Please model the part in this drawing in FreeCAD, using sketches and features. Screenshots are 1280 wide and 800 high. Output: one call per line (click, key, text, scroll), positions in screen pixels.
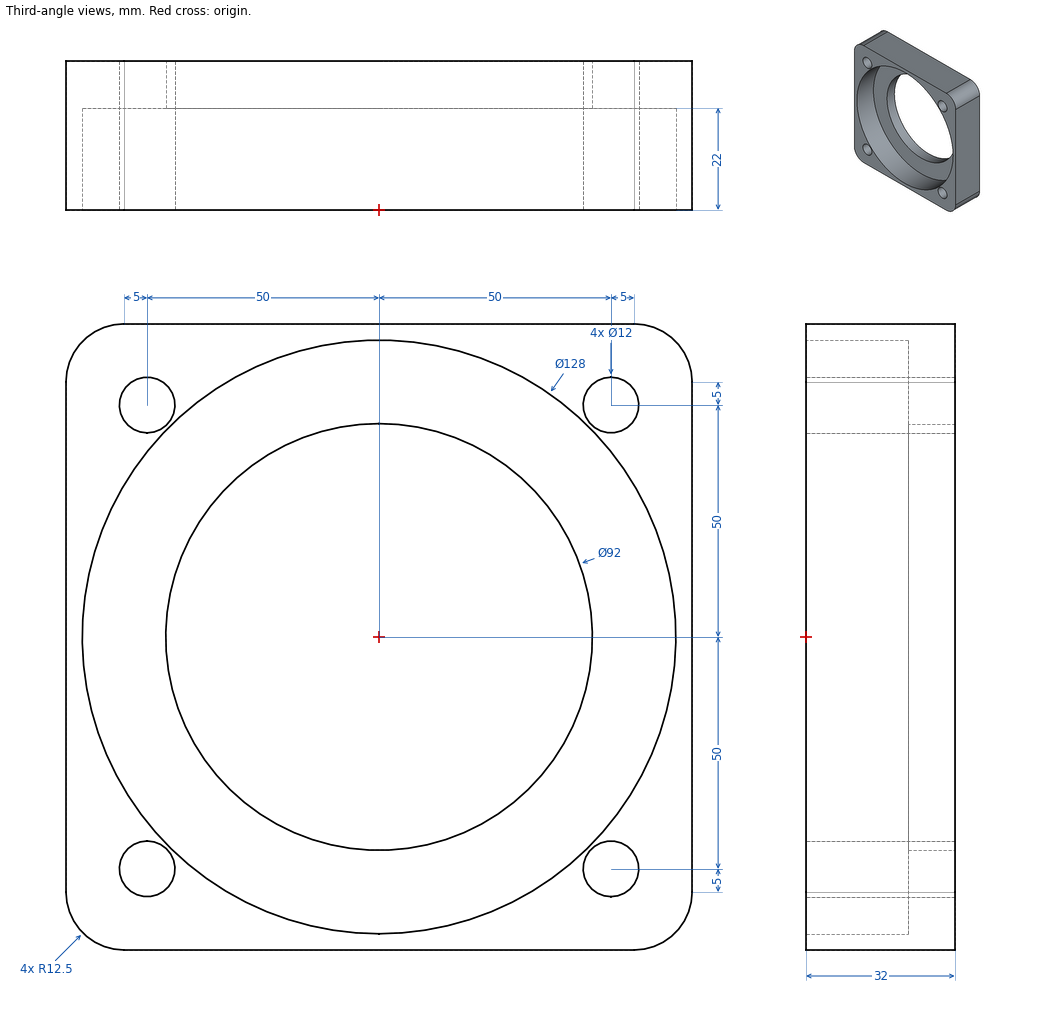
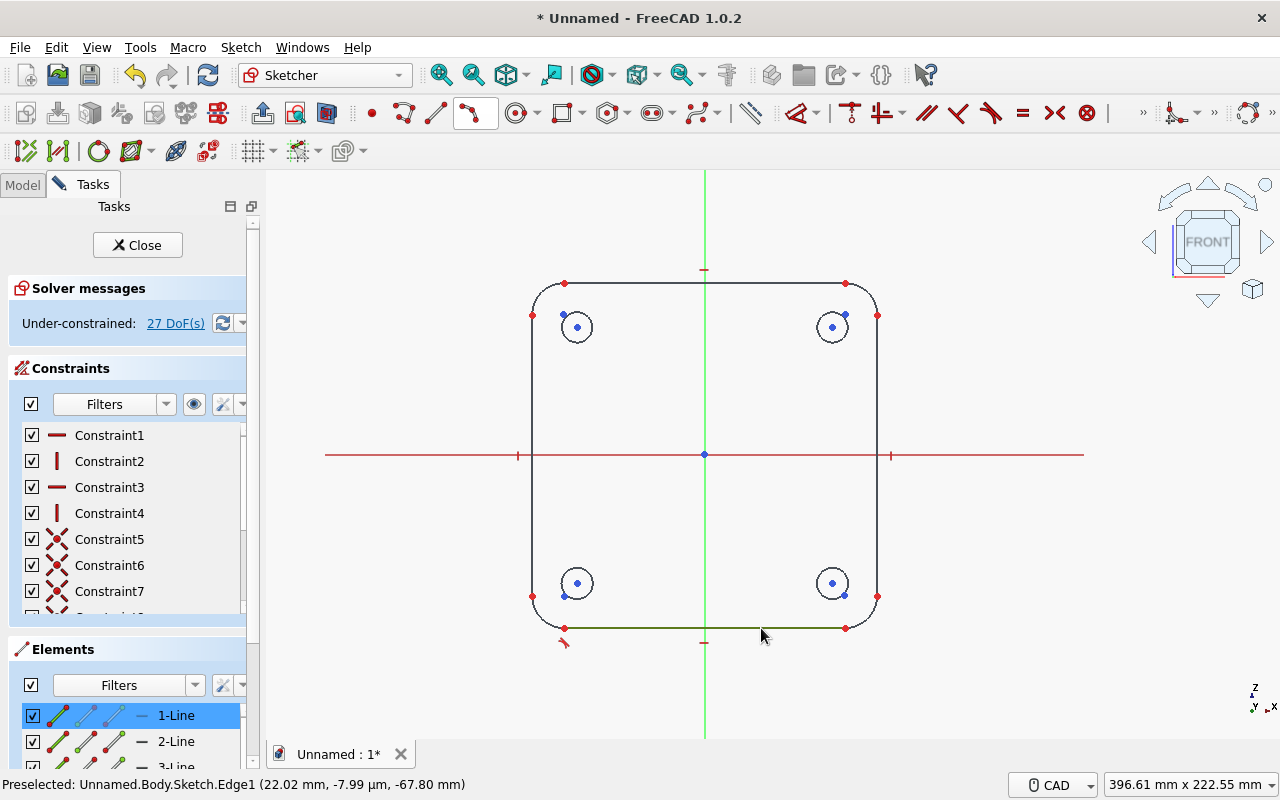
click(860, 624)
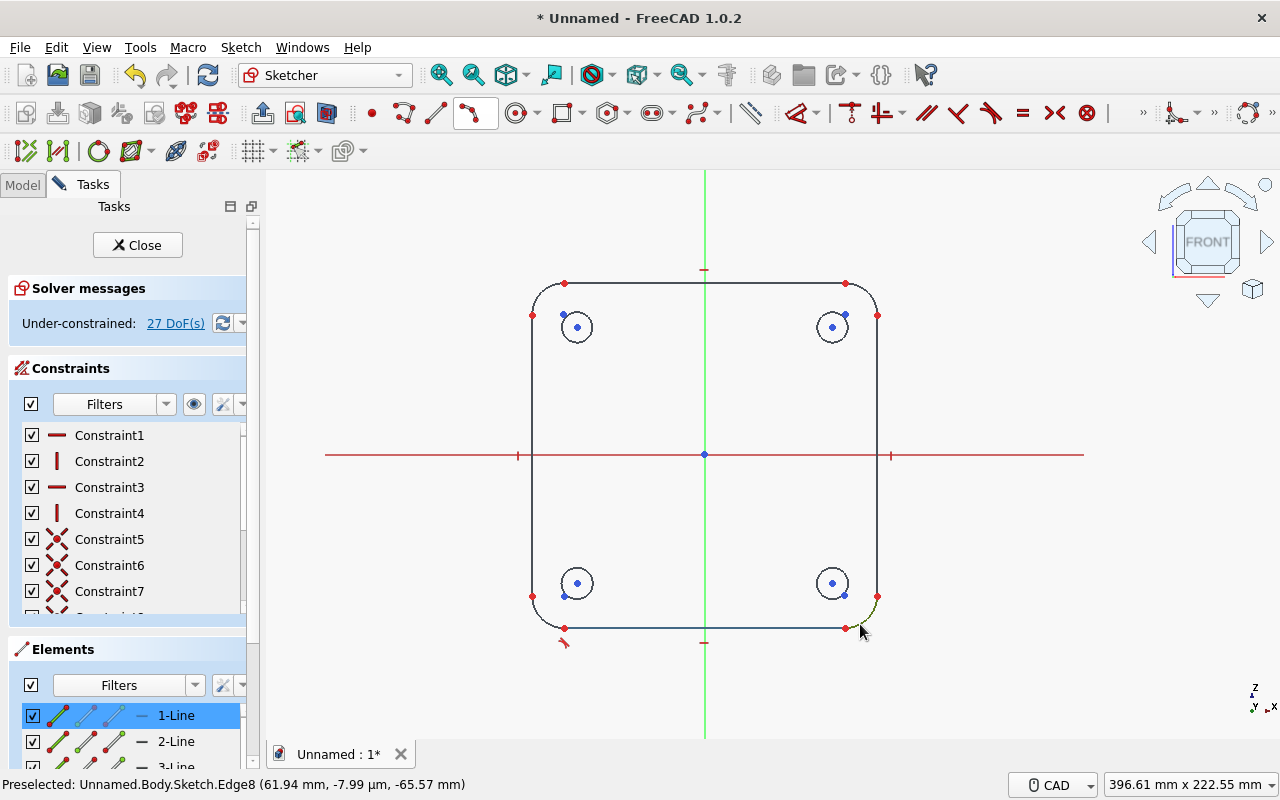
click(992, 114)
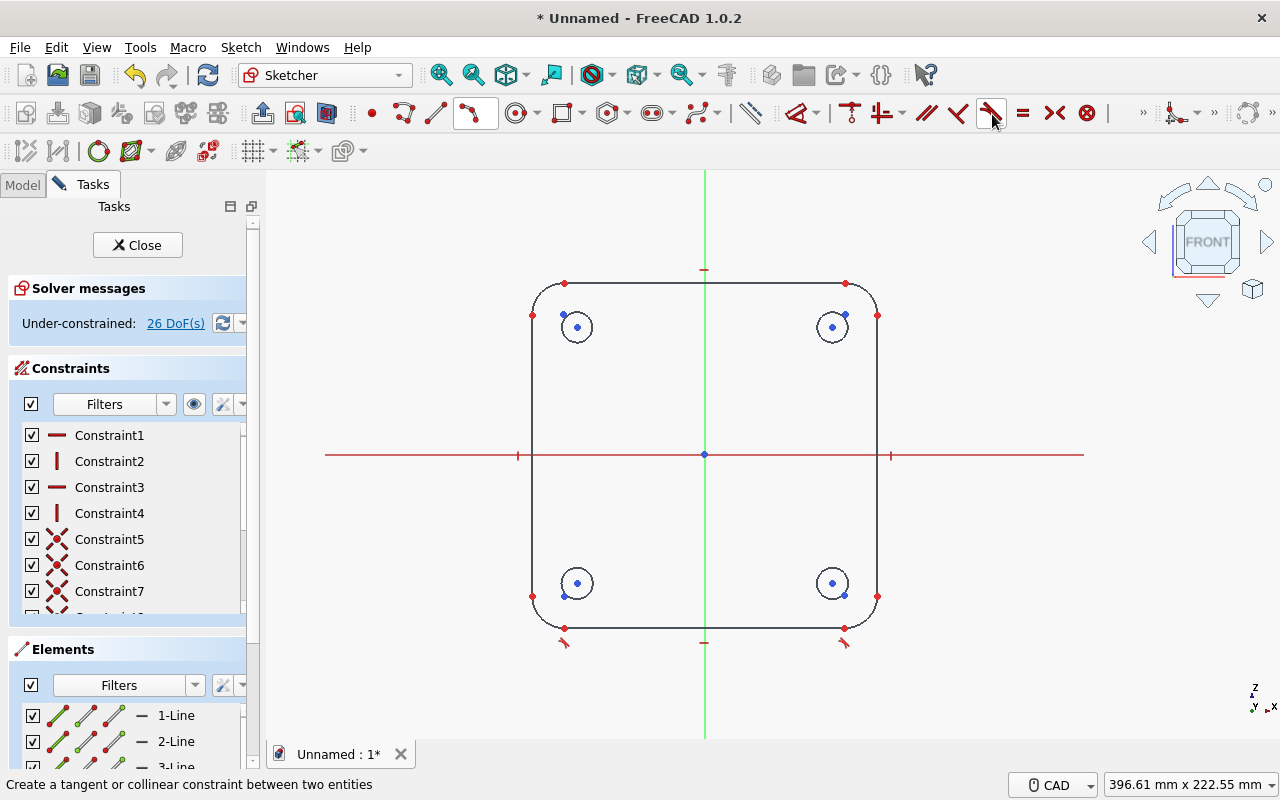
click(532, 512)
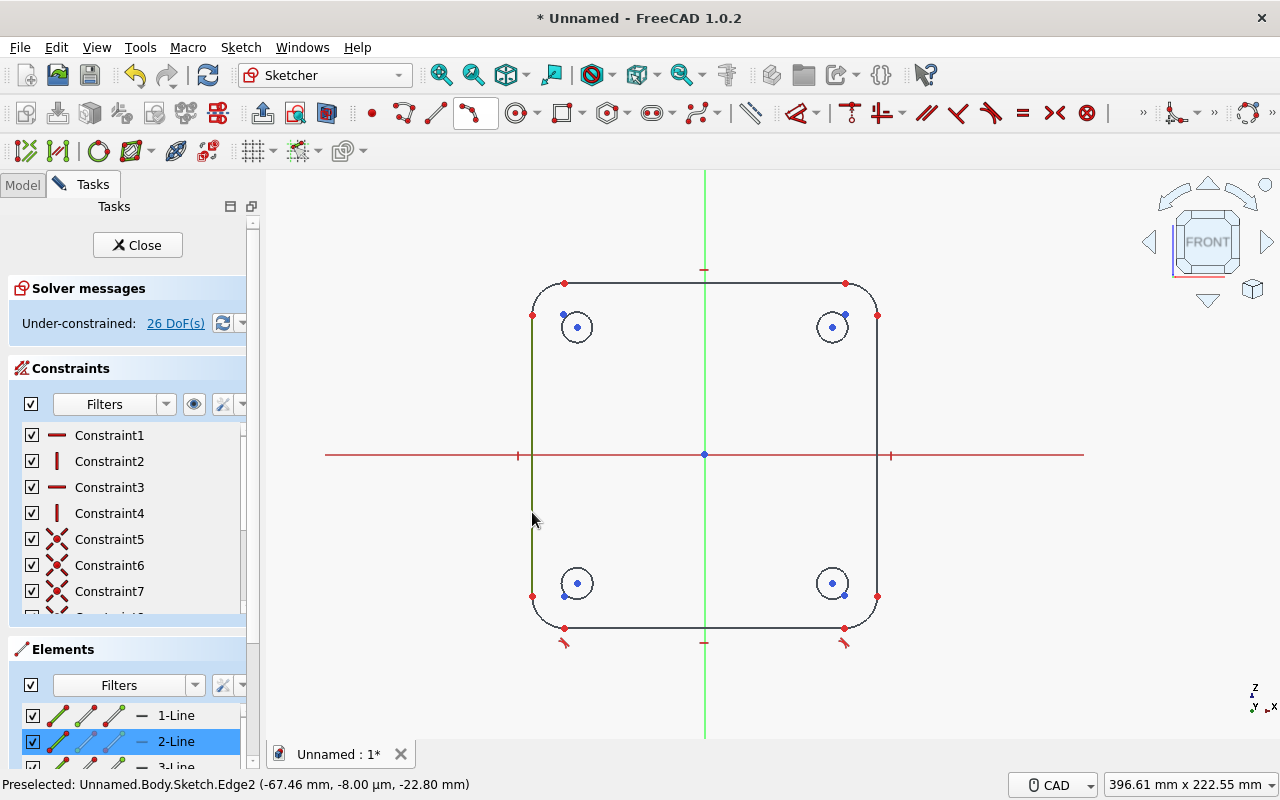
click(536, 611)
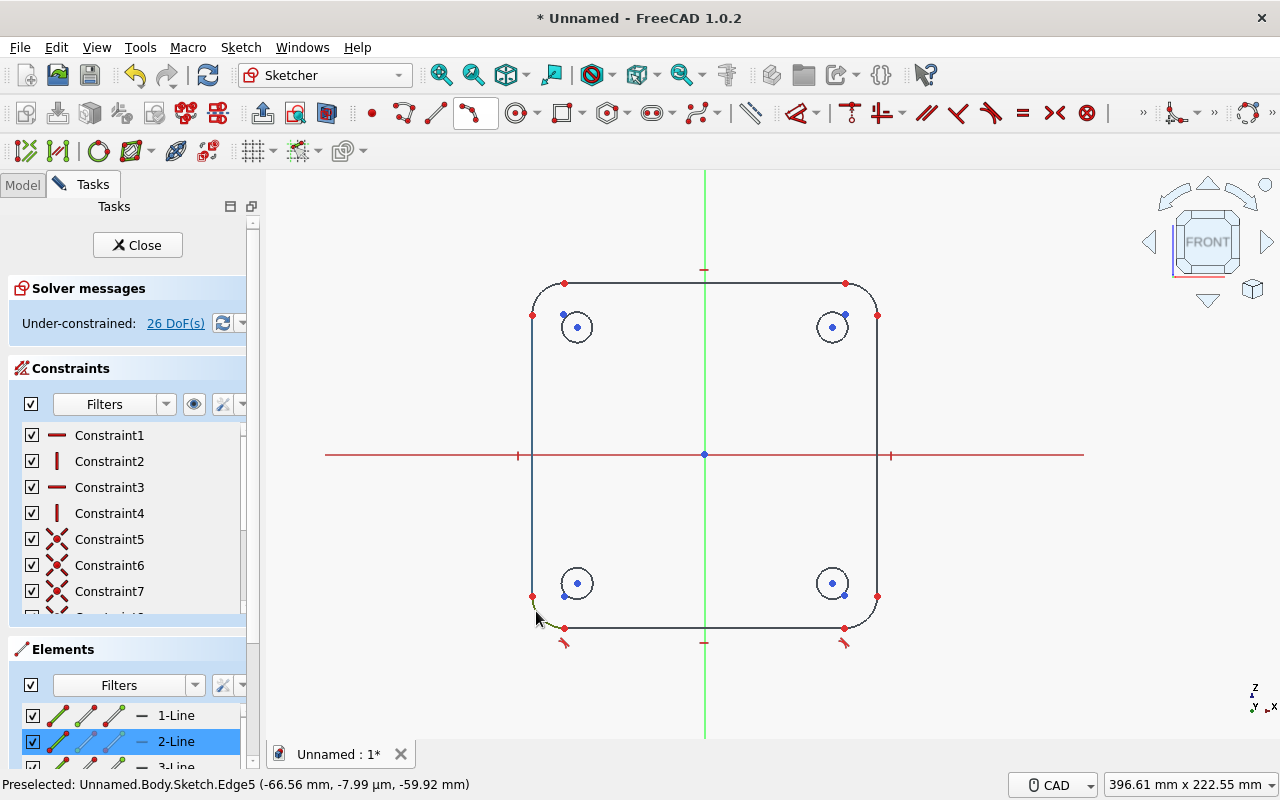
click(992, 114)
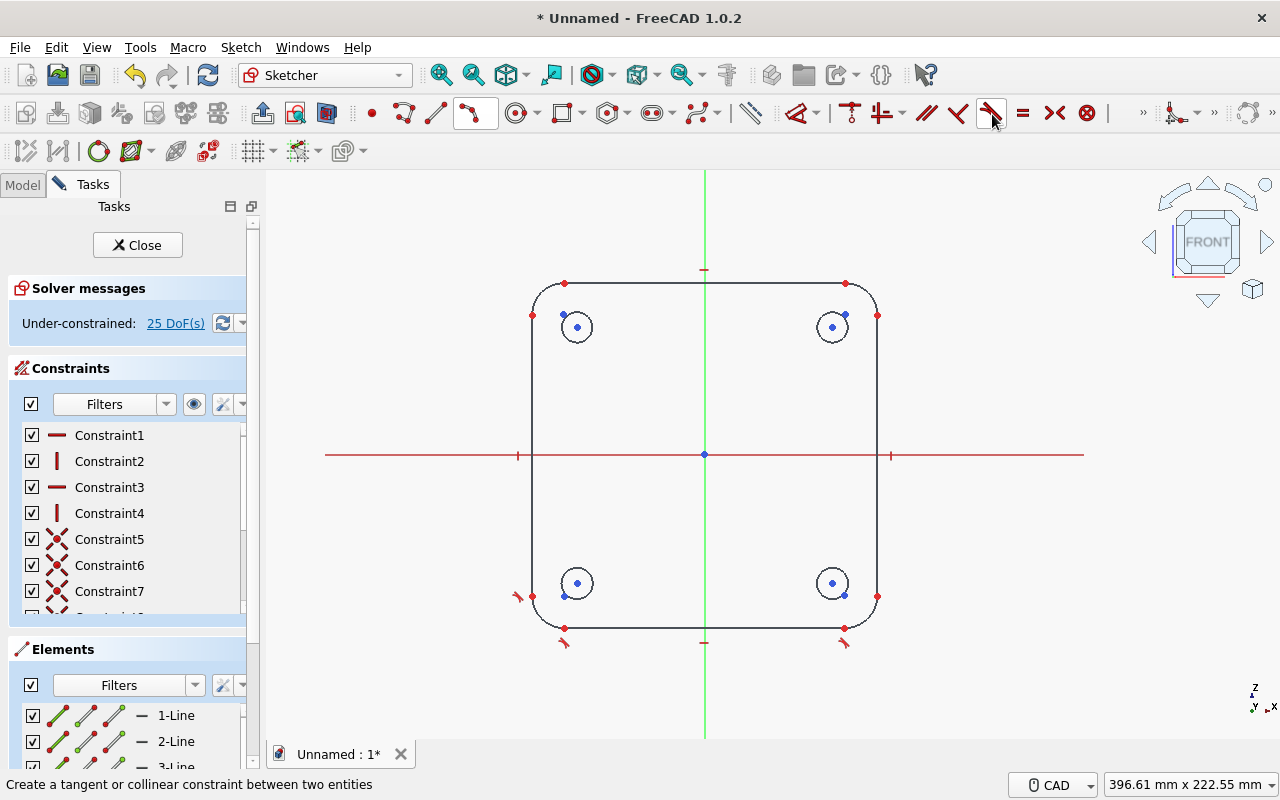
click(532, 512)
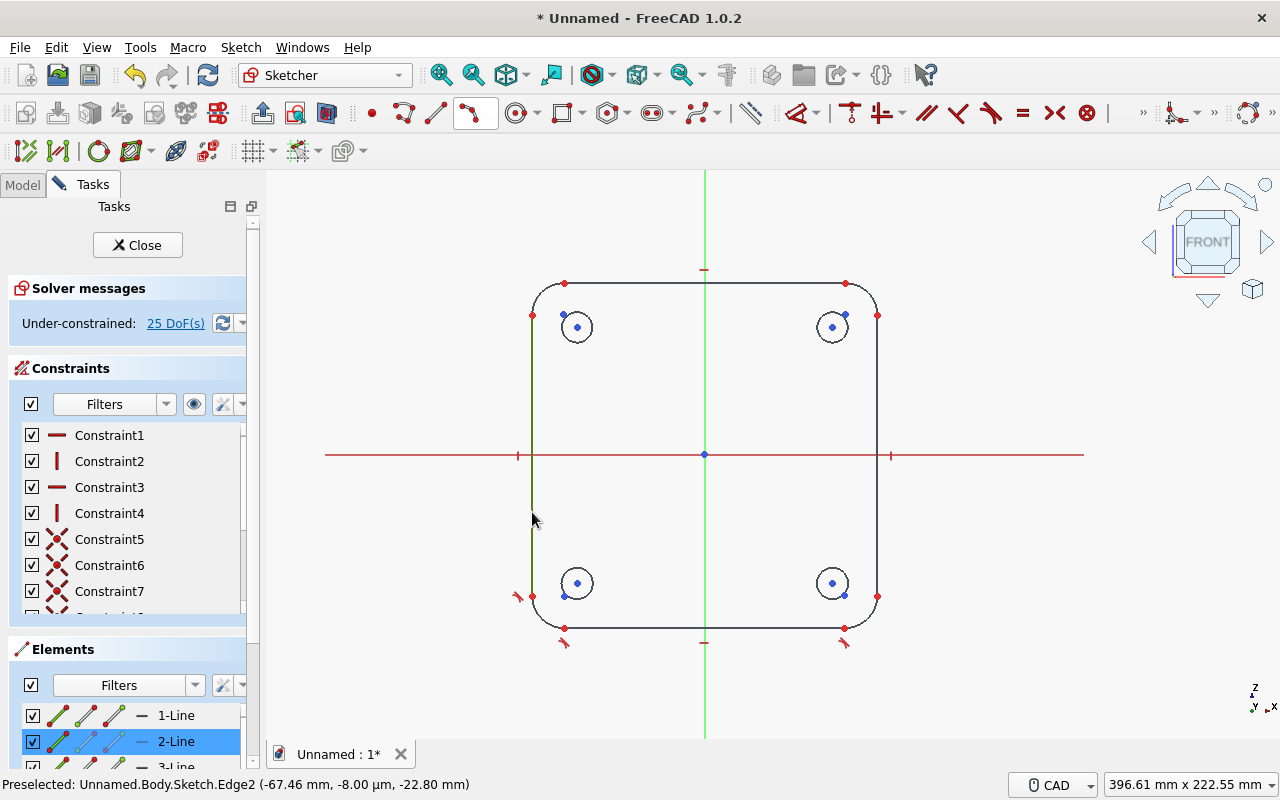
click(550, 287)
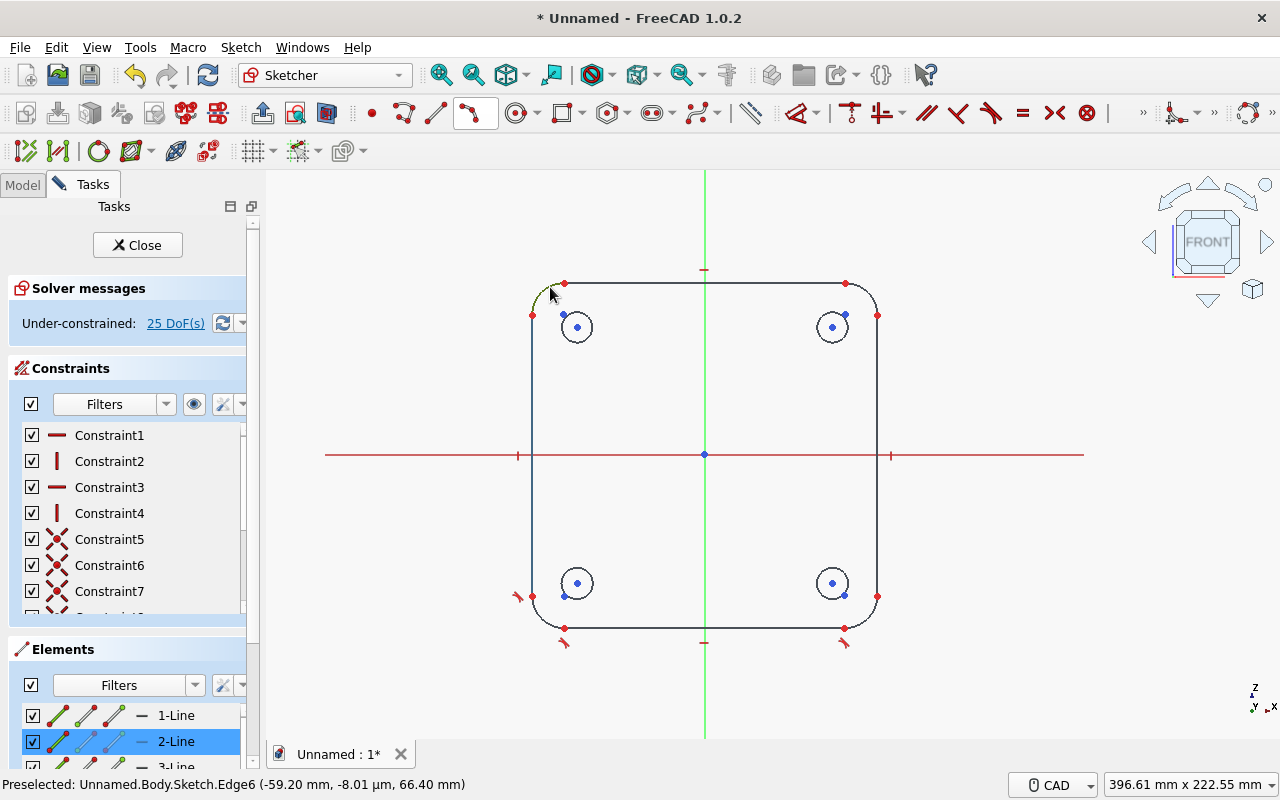
key(t)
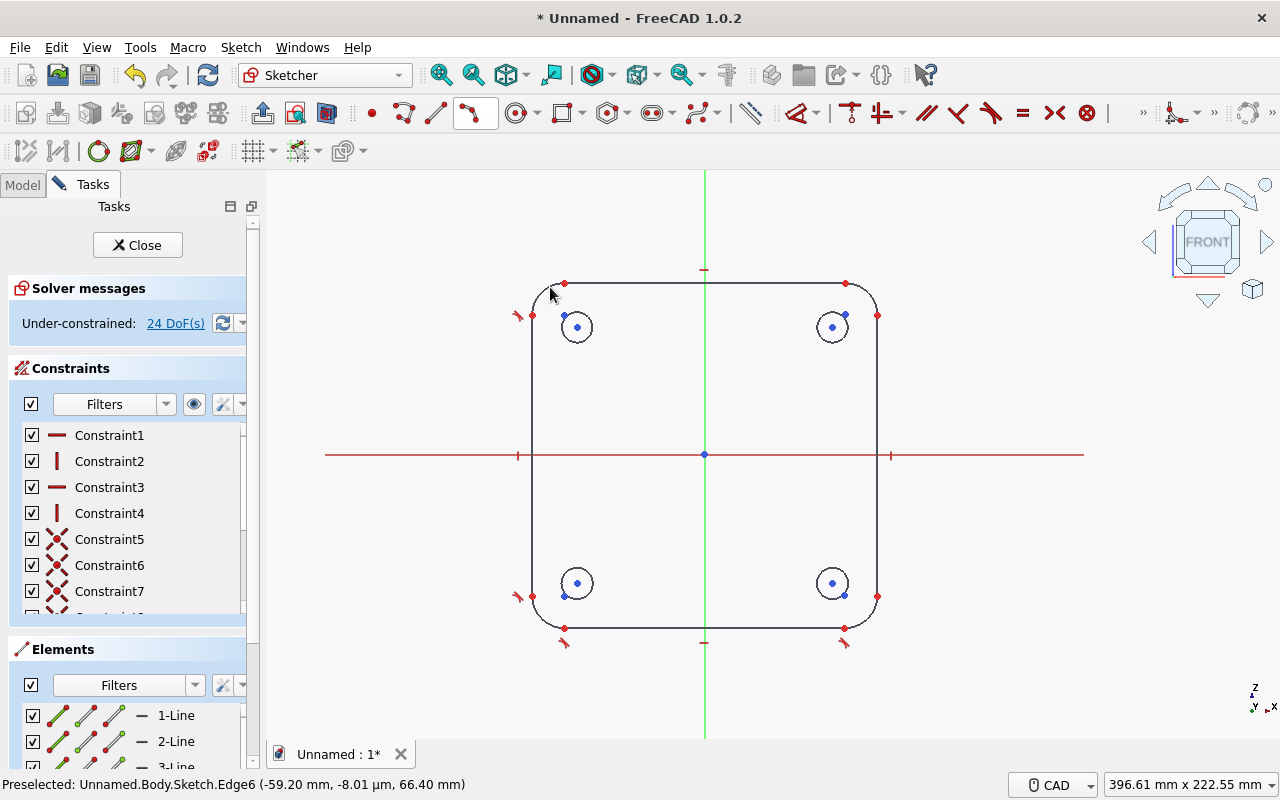
click(649, 283)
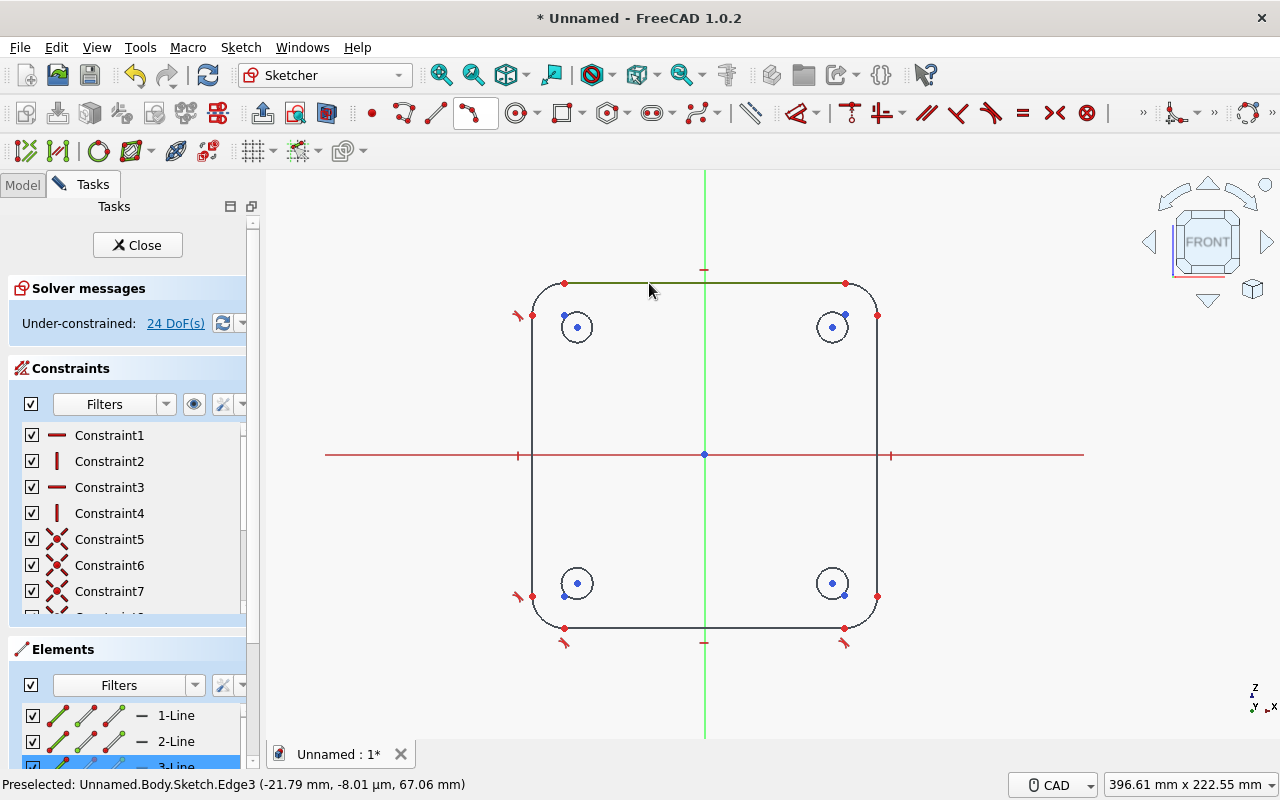
click(550, 287)